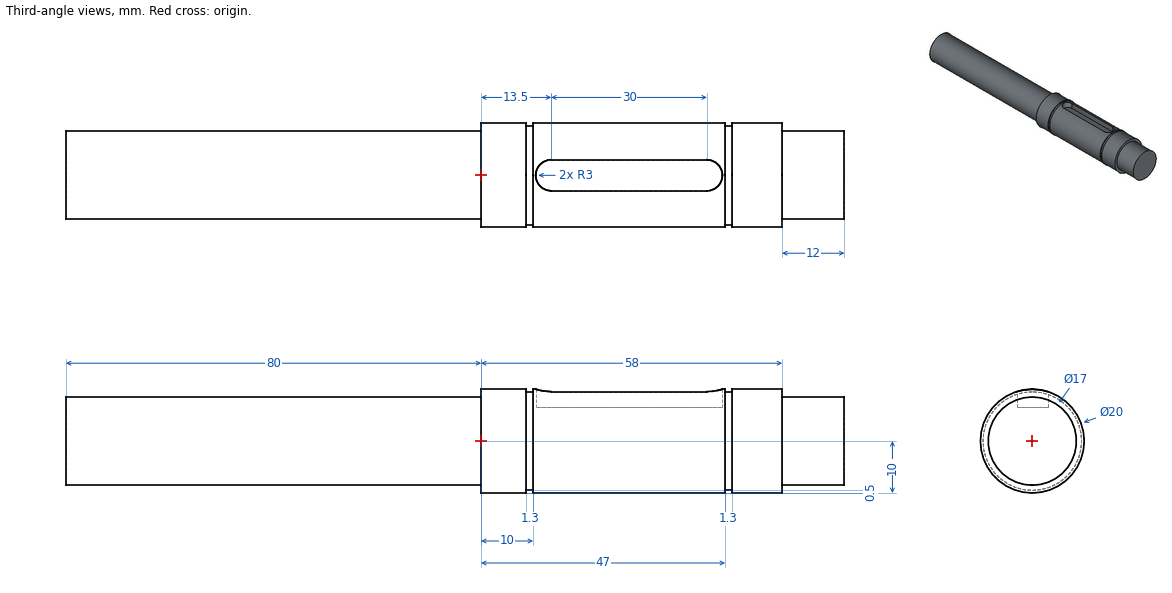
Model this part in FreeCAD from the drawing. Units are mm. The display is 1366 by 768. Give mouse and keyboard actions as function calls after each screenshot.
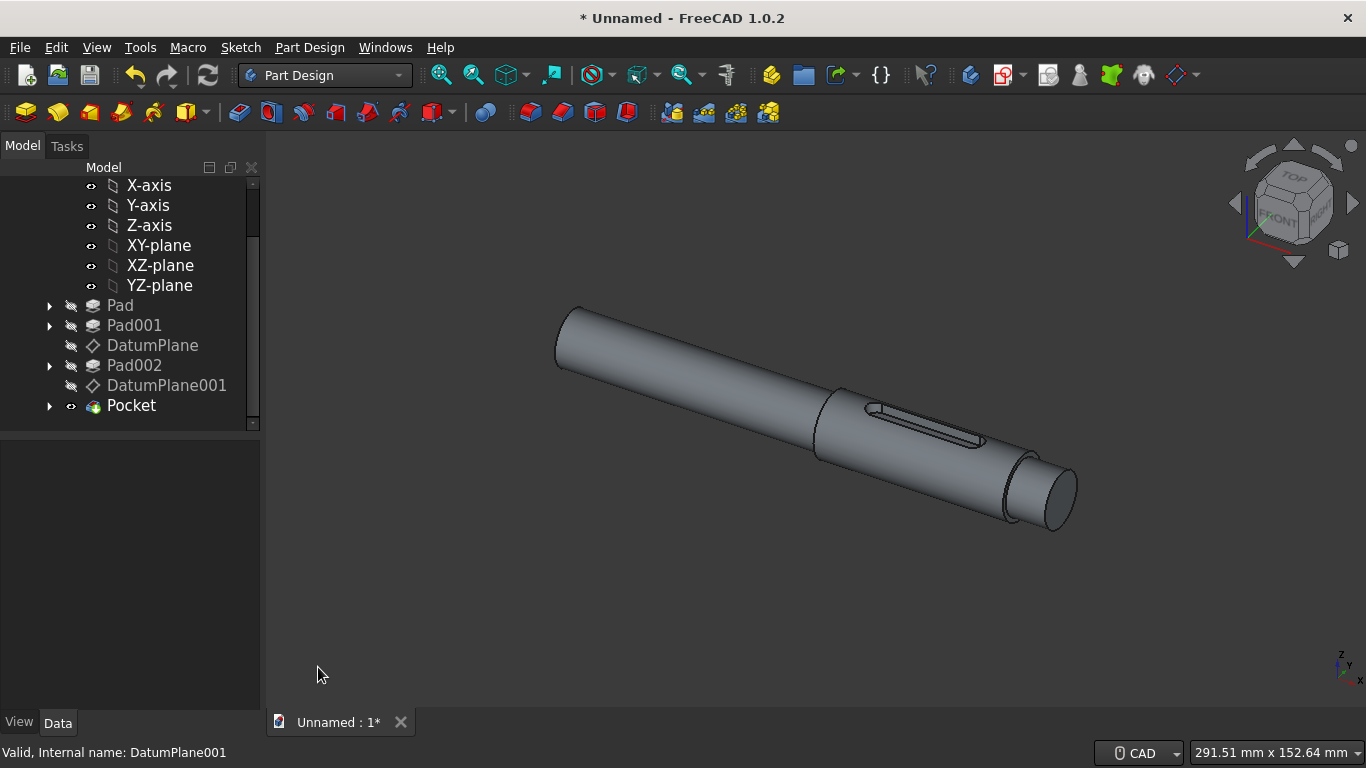
click(1004, 76)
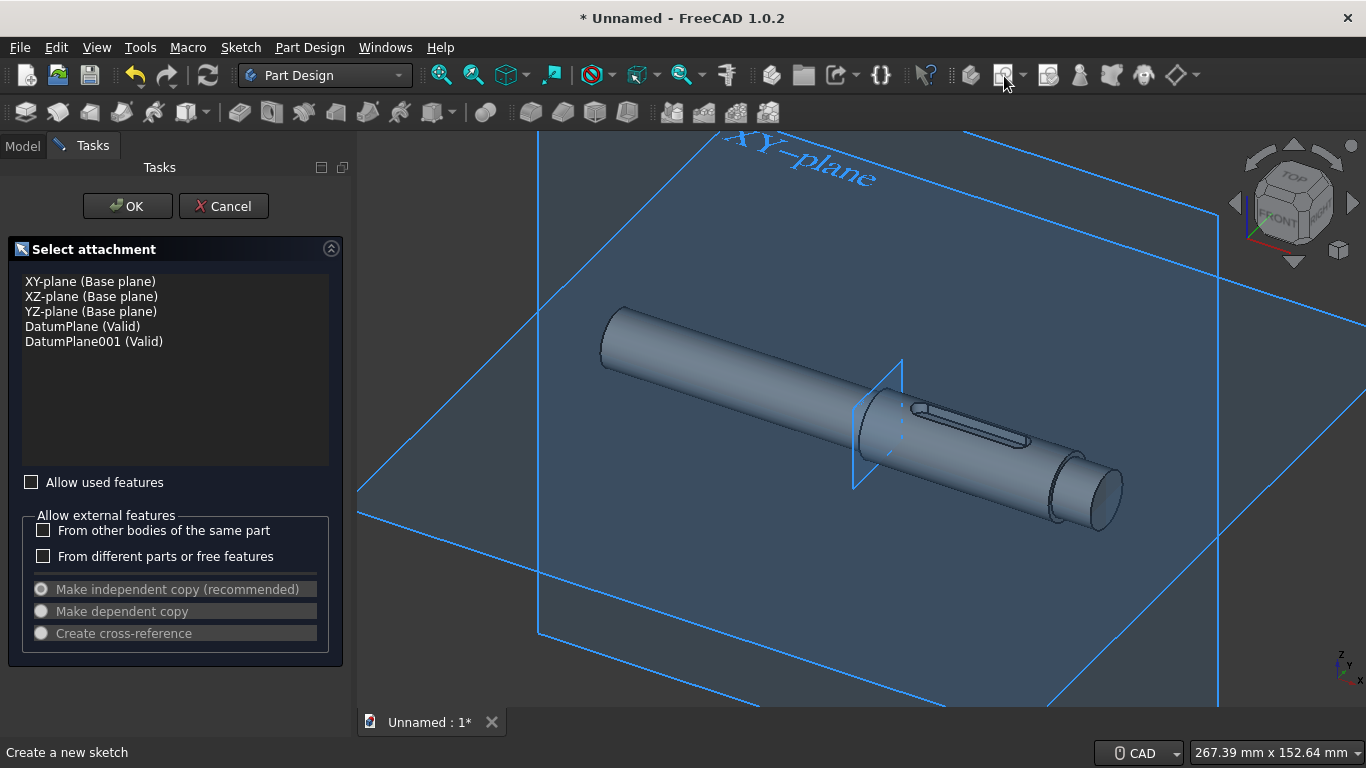
click(82, 296)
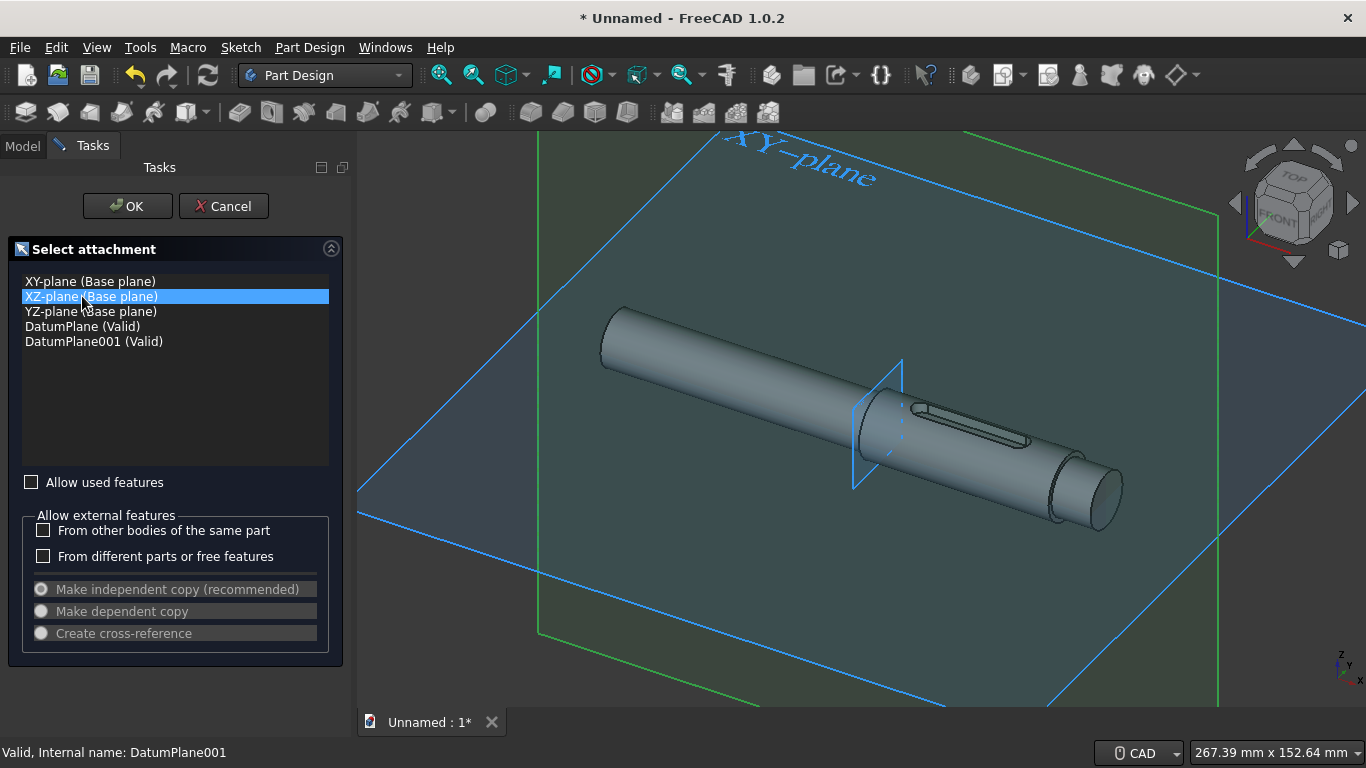
click(128, 206)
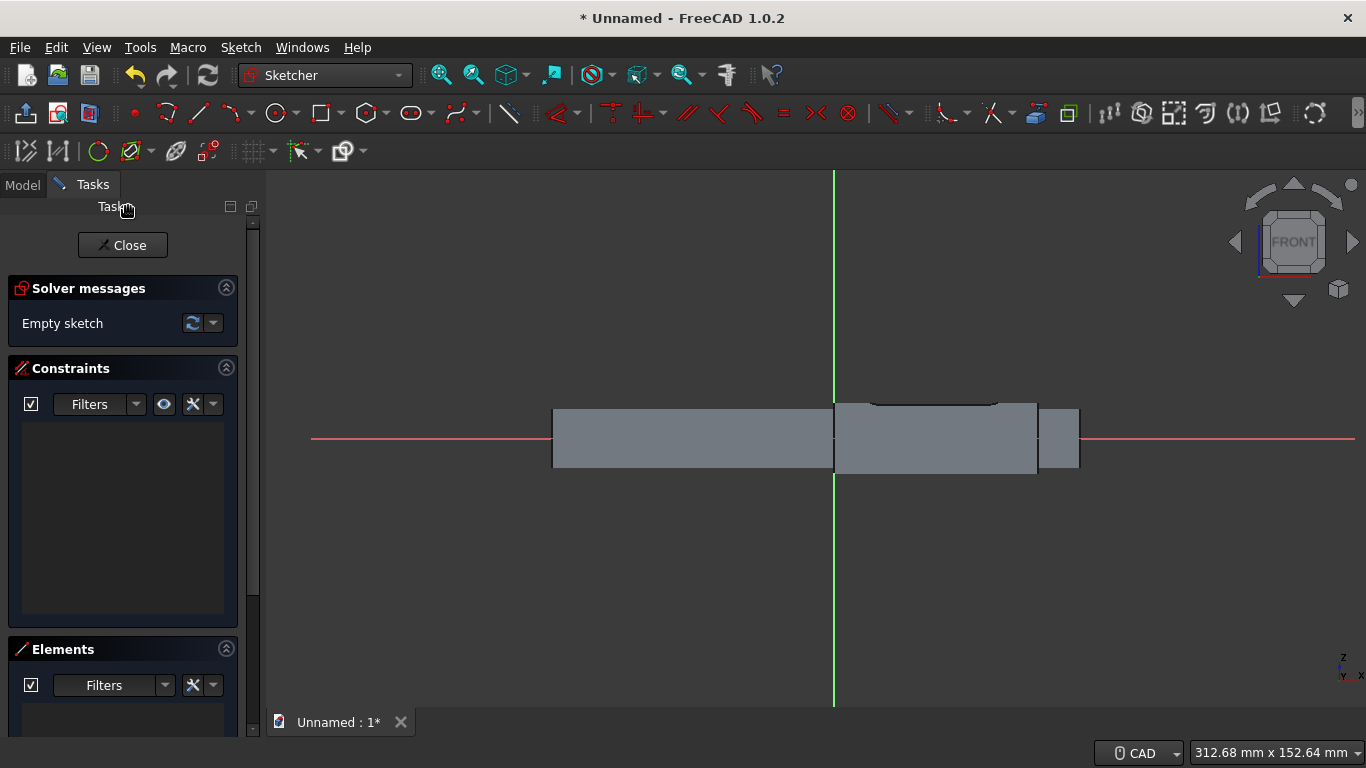
key(q)
key(s)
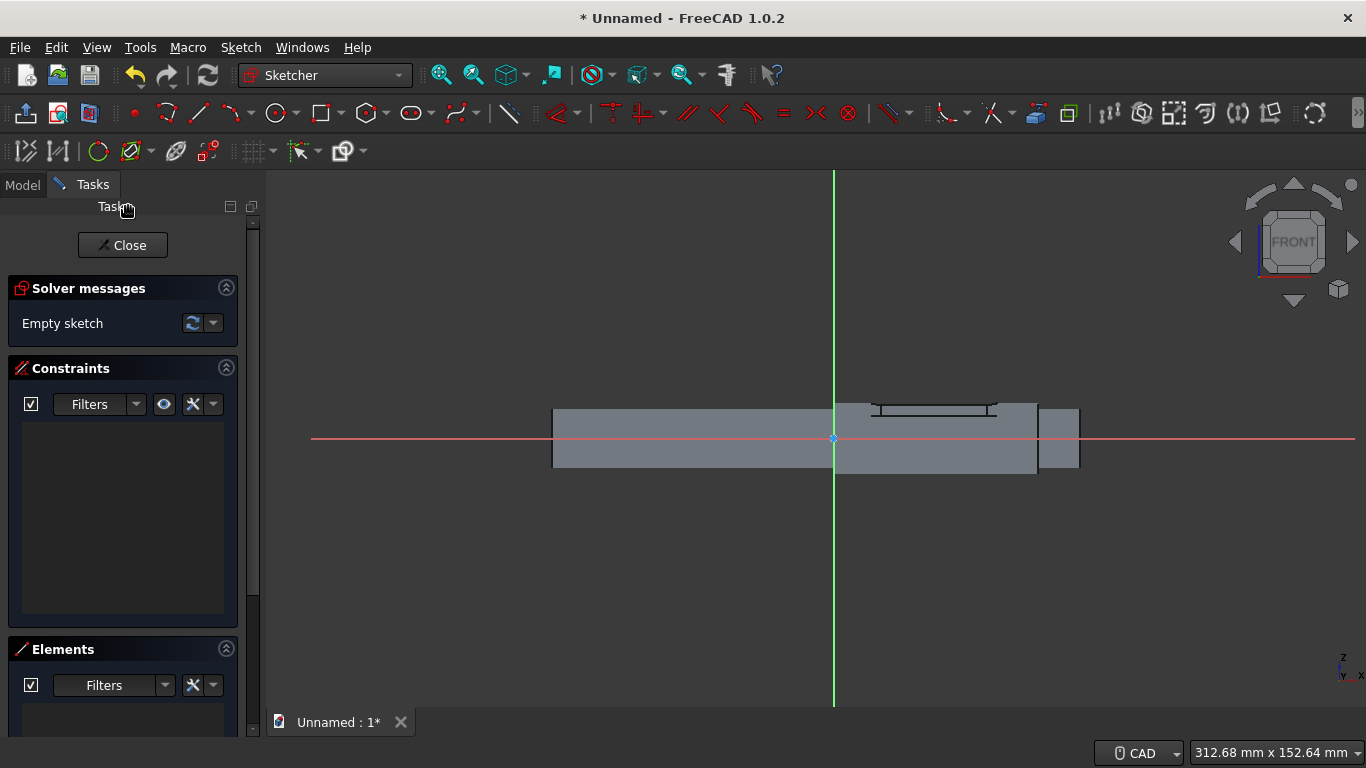
scroll(975, 462, up, 7)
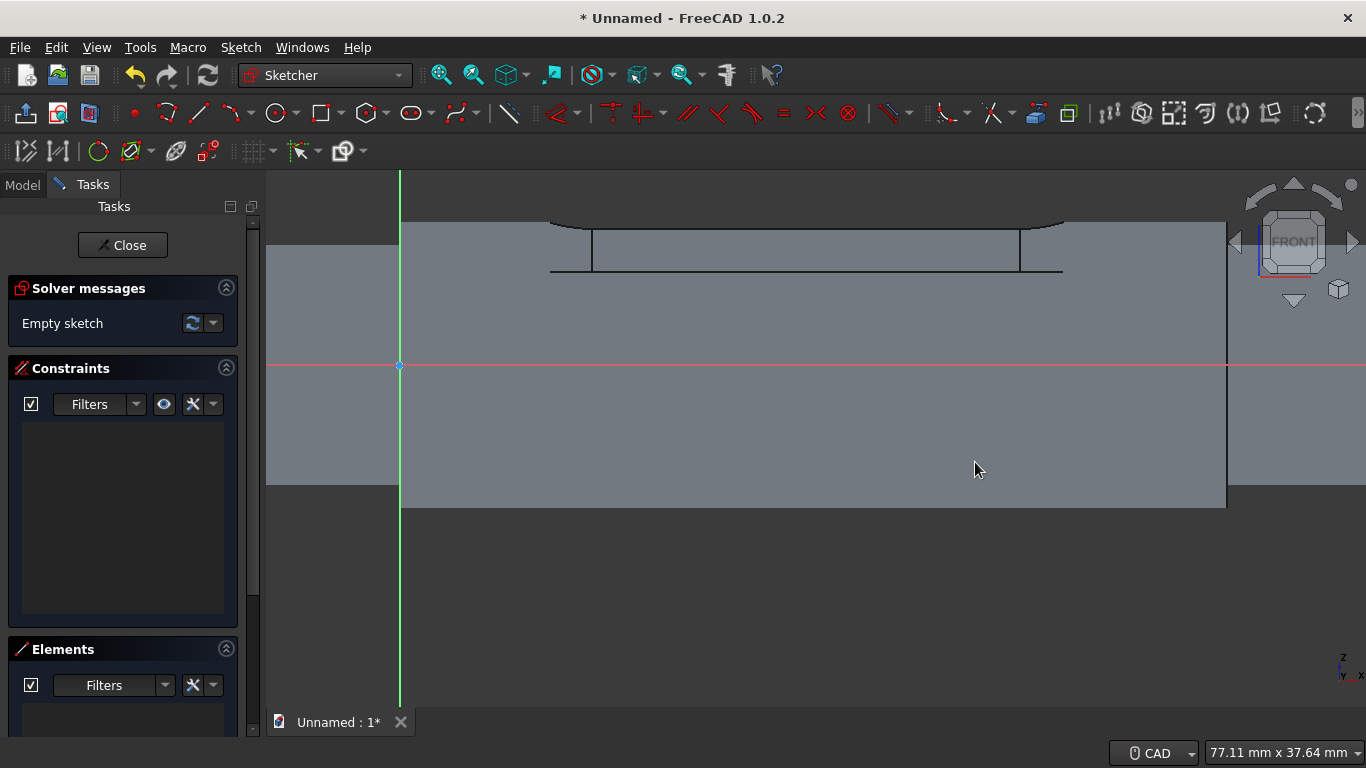
key(g)
key(r)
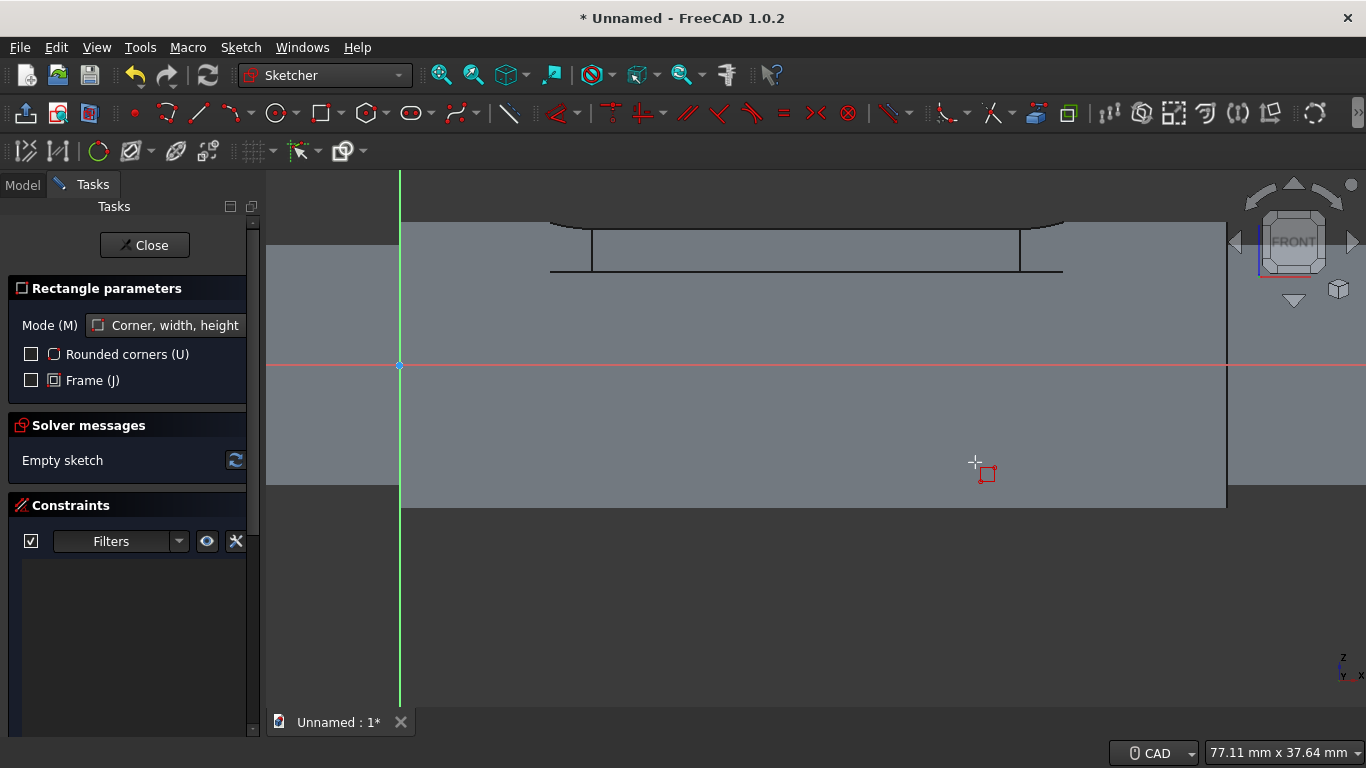
scroll(524, 501, up, 5)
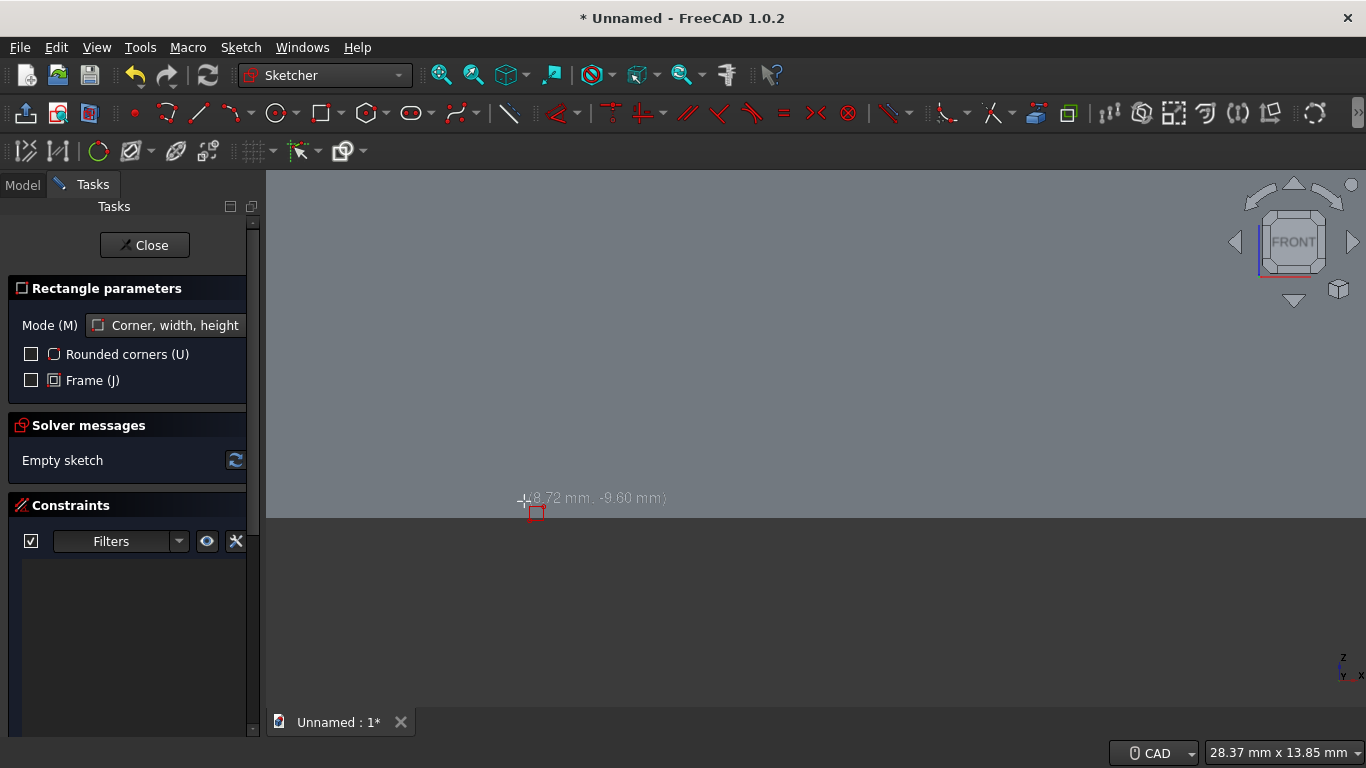
click(523, 499)
click(573, 518)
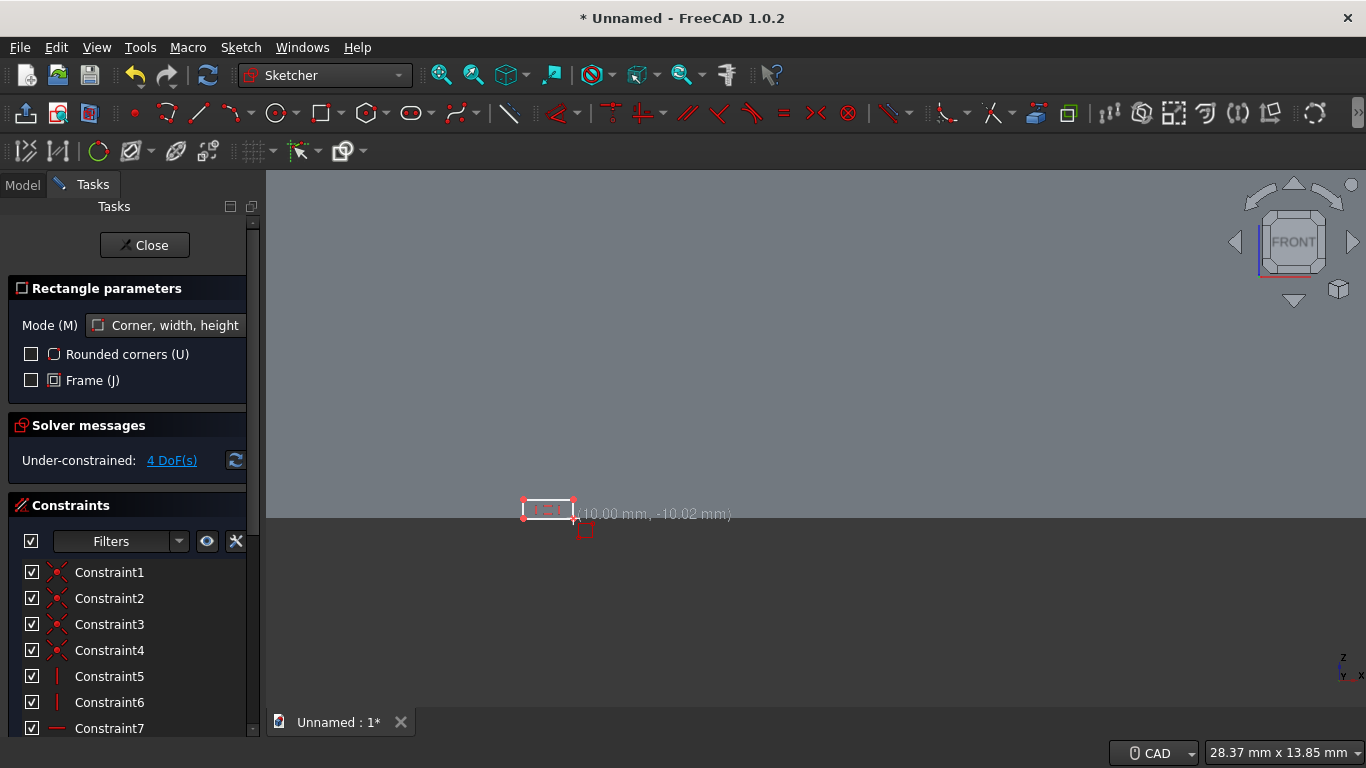
scroll(530, 505, down, 5)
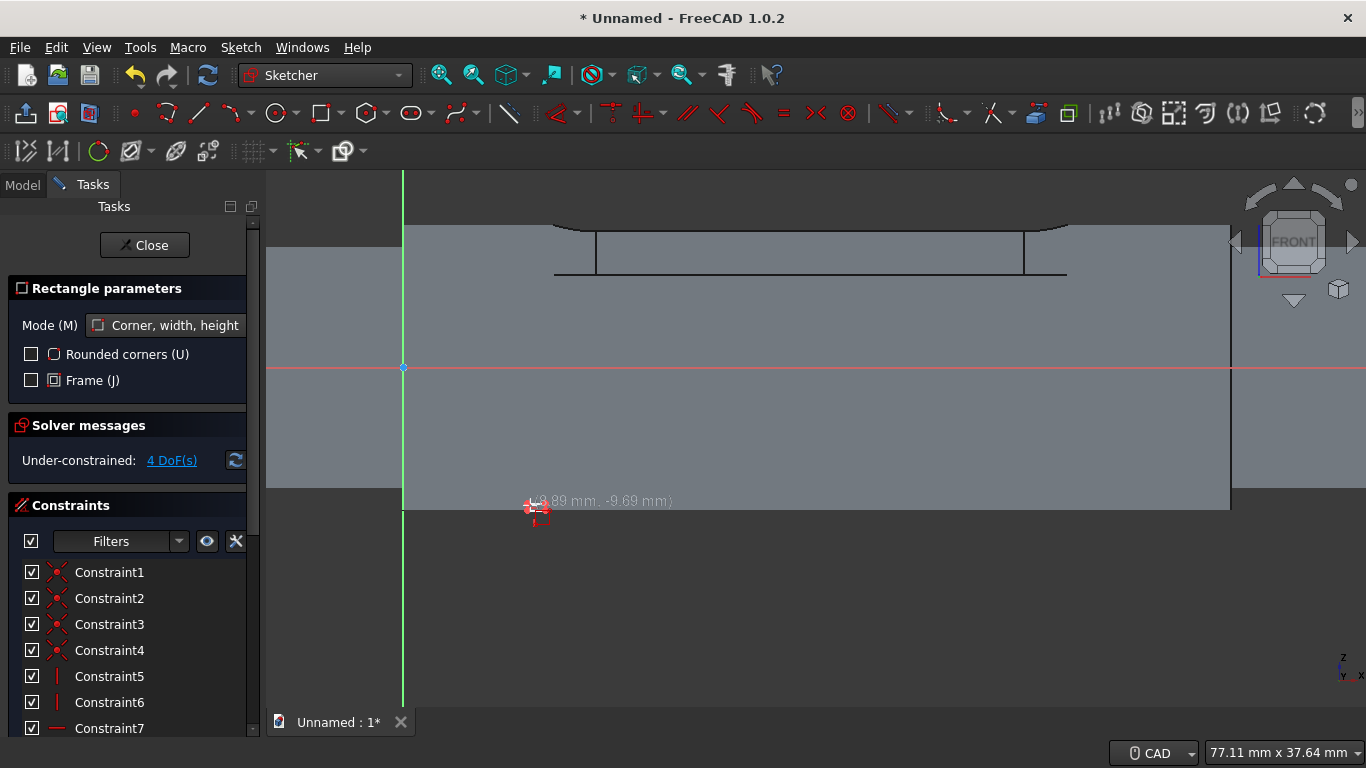
scroll(1074, 503, up, 5)